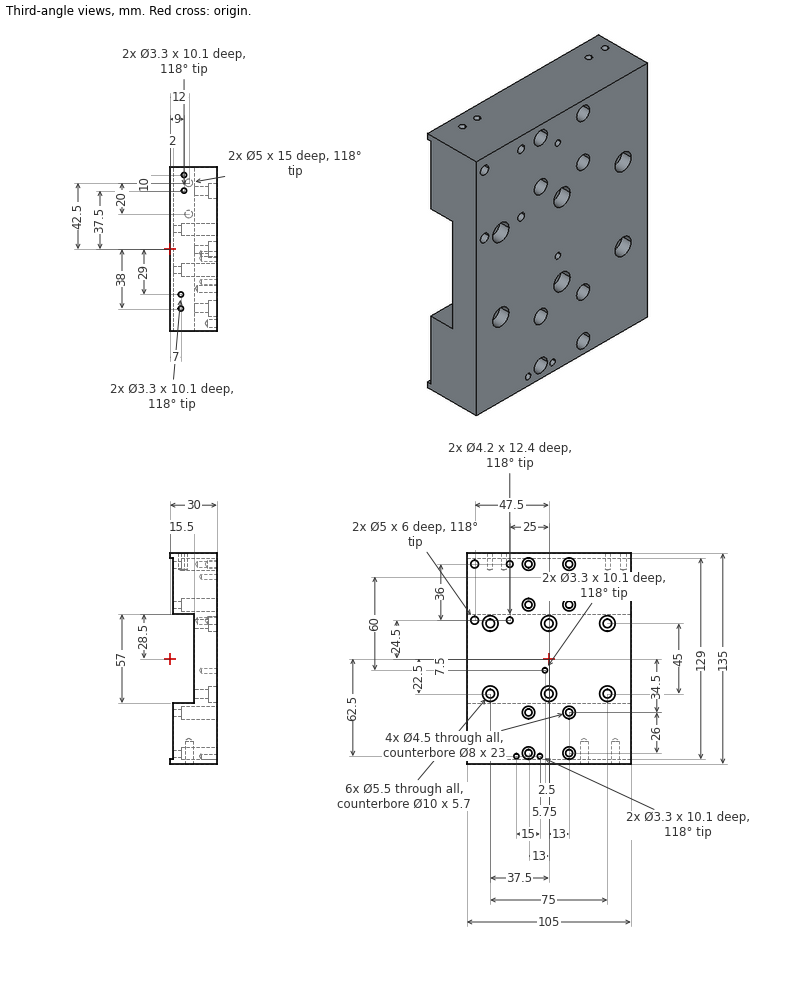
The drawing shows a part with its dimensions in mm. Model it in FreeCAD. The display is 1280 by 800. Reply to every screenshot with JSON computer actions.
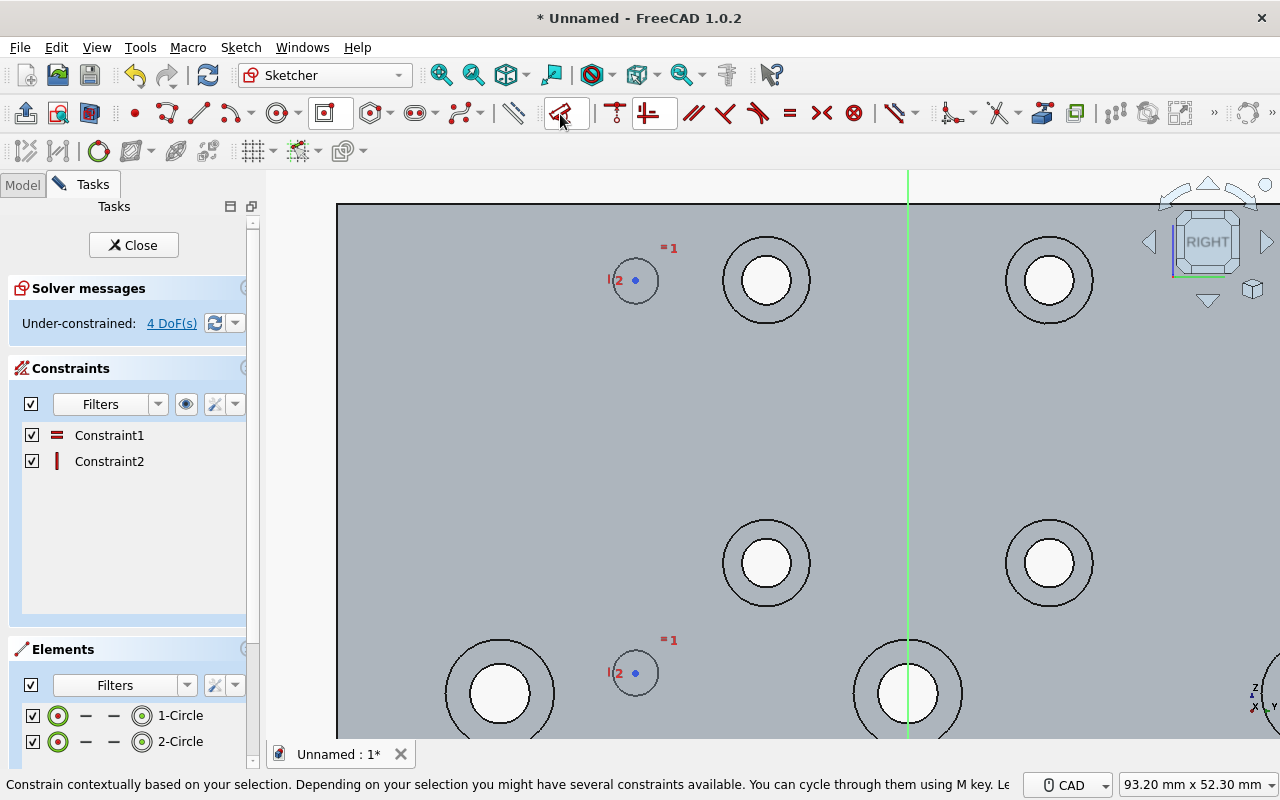
{"action": "left_click", "coordinate": [652, 657]}
{"action": "left_click", "coordinate": [675, 634]}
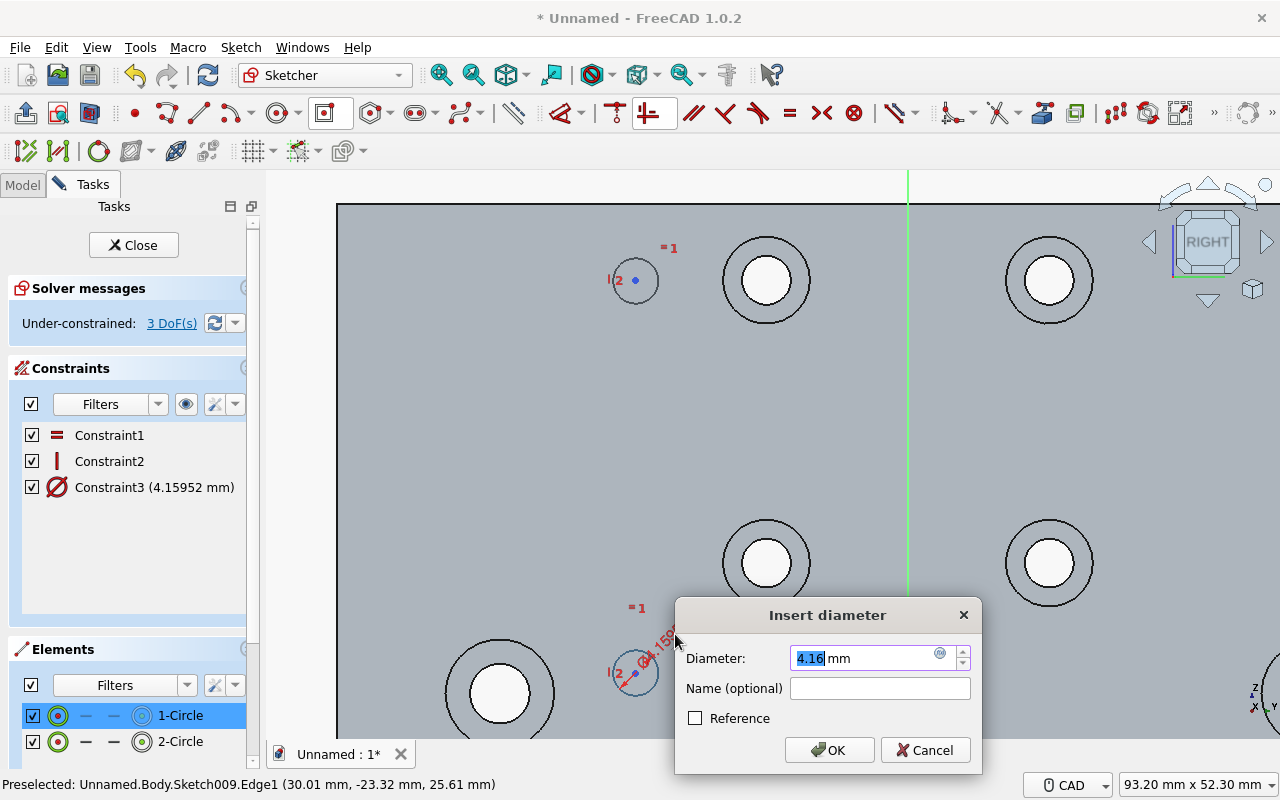
{"action": "type", "text": "4.2"}
{"action": "key", "text": "Return"}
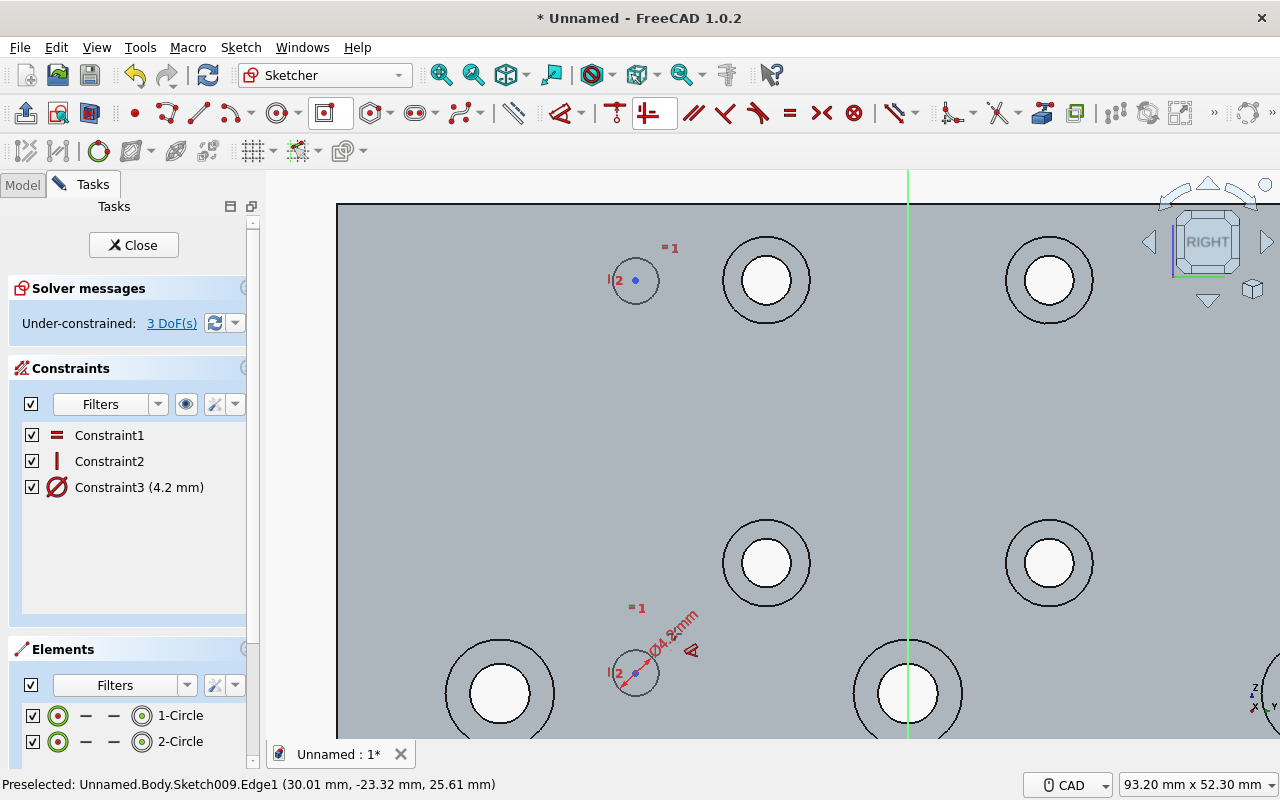
{"action": "left_click", "coordinate": [636, 673]}
{"action": "left_click", "coordinate": [772, 639]}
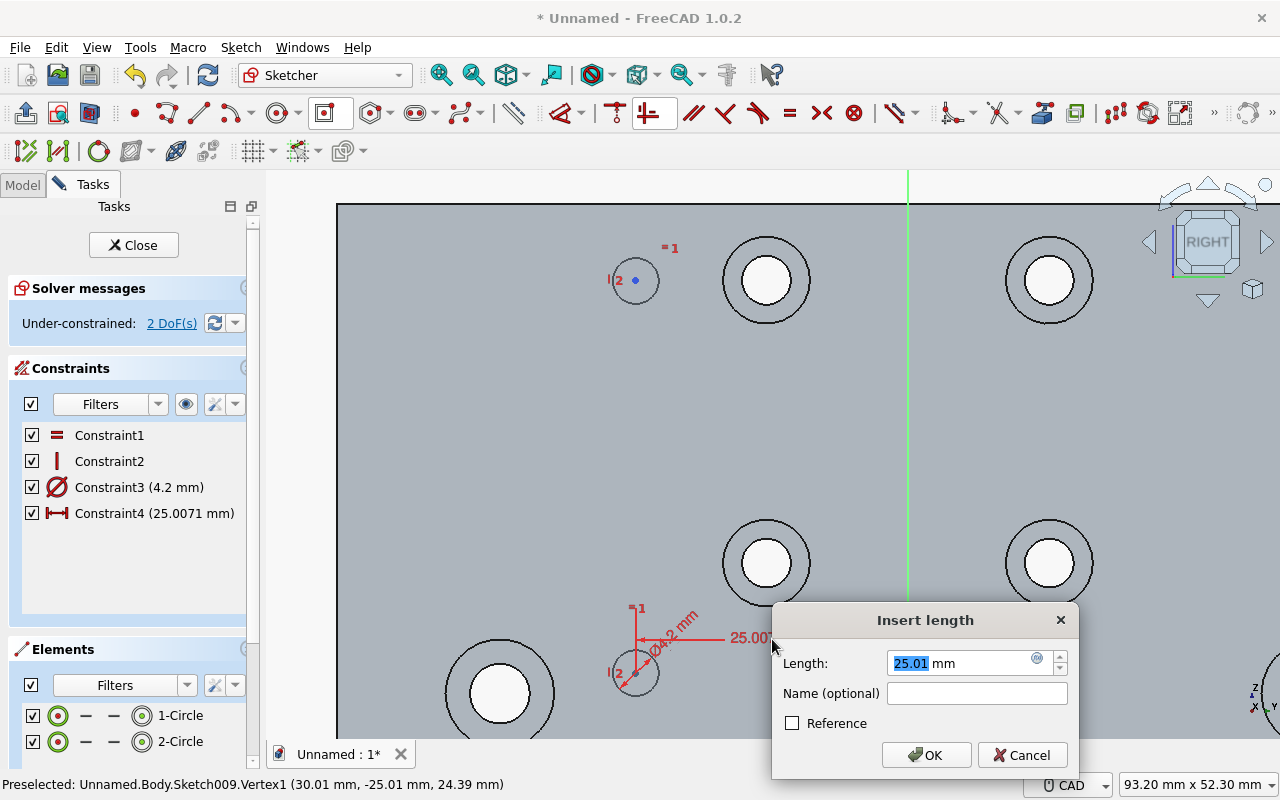
{"action": "type", "text": "25"}
{"action": "key", "text": "Return"}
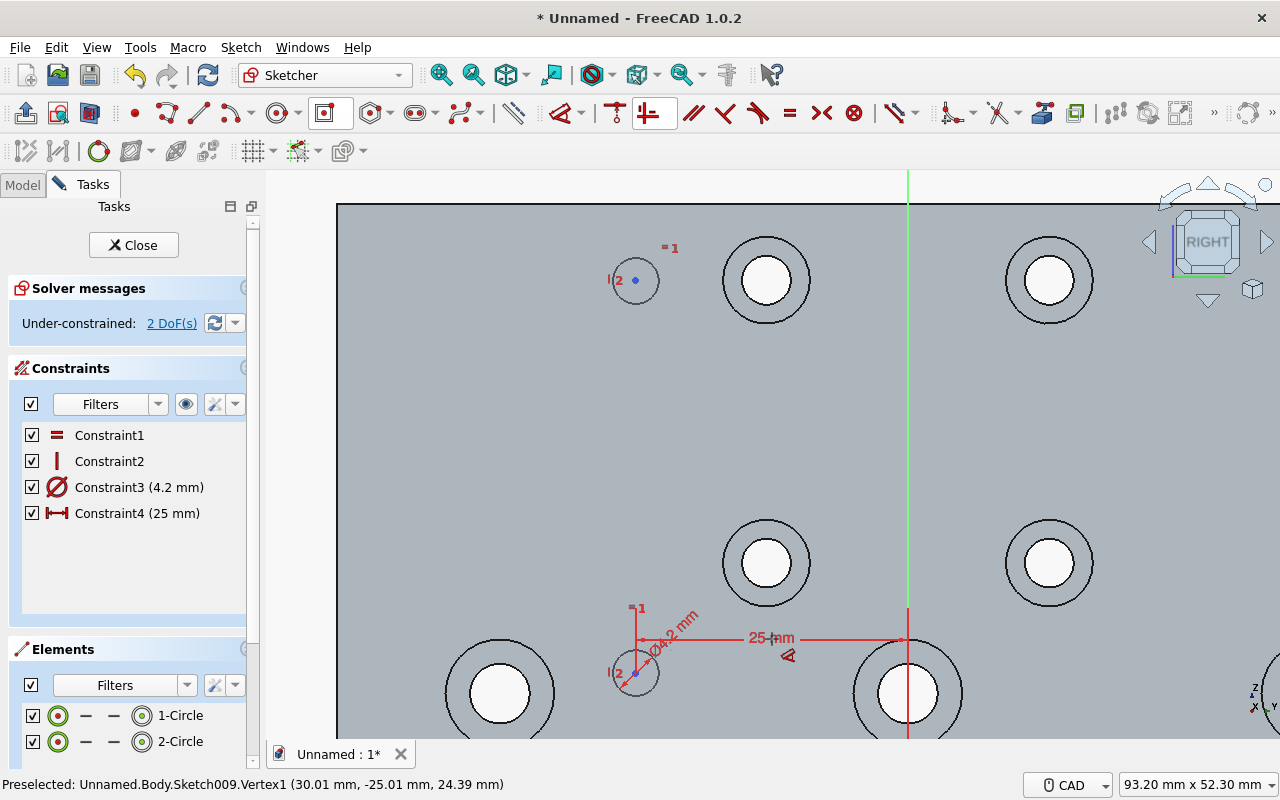
{"action": "left_click", "coordinate": [636, 673]}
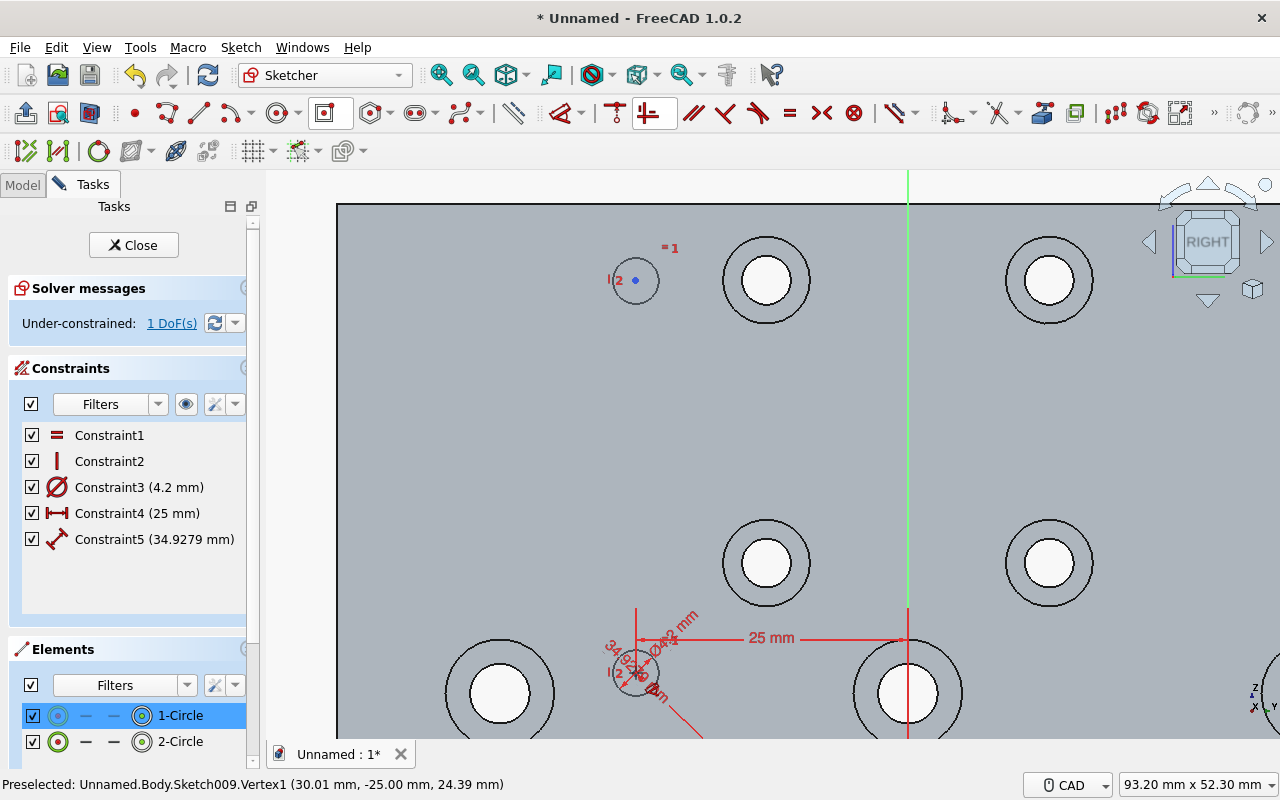
{"action": "left_click", "coordinate": [636, 281]}
{"action": "left_click", "coordinate": [602, 477]}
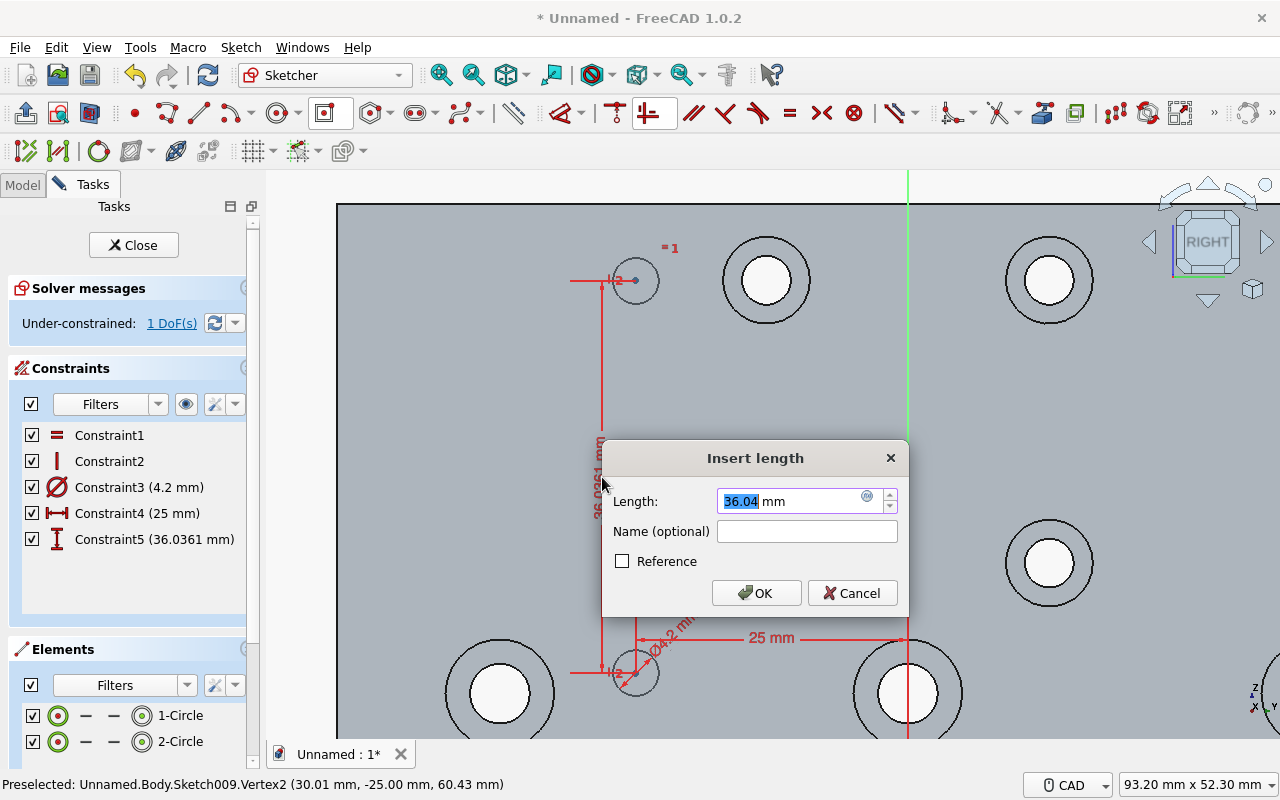
{"action": "type", "text": "36"}
{"action": "key", "text": "Return"}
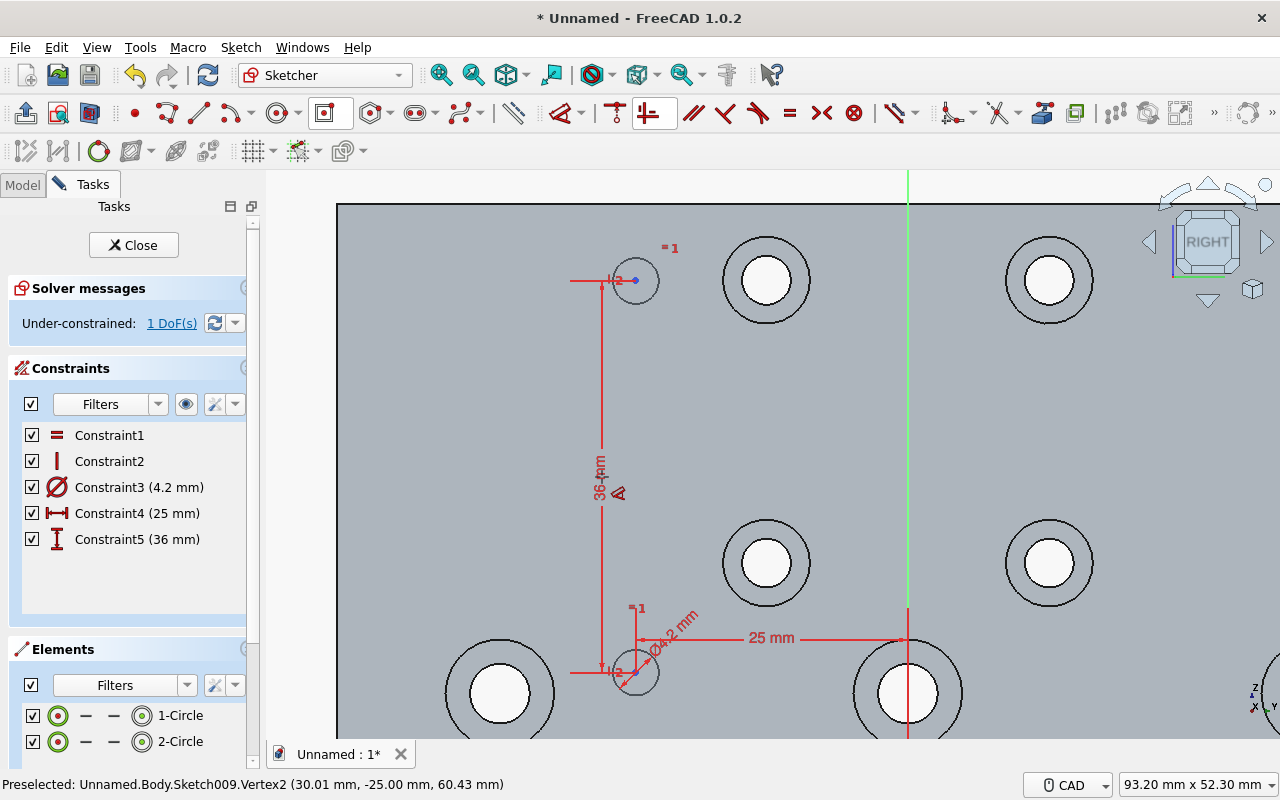
{"action": "left_click", "coordinate": [636, 673]}
{"action": "left_click", "coordinate": [942, 692]}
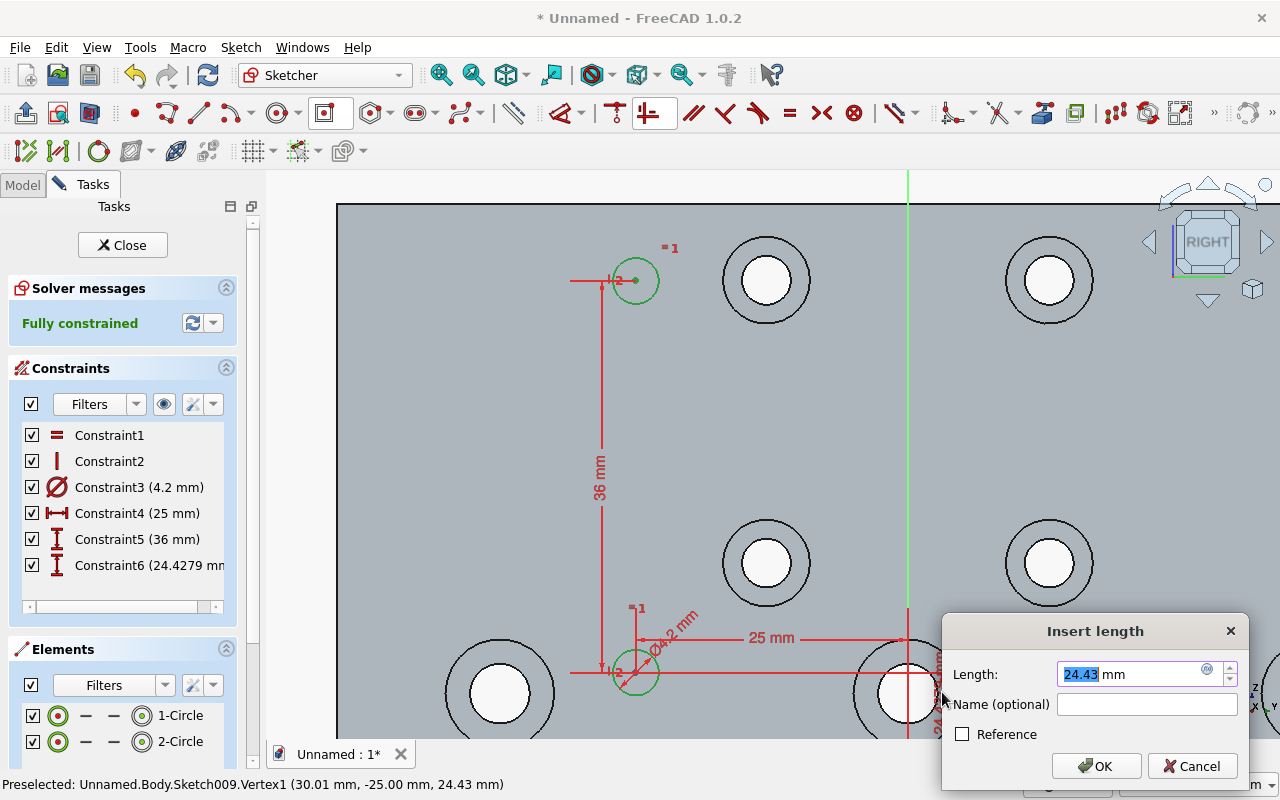
{"action": "type", "text": "24.5"}
{"action": "key", "text": "Return"}
{"action": "key", "text": "Escape"}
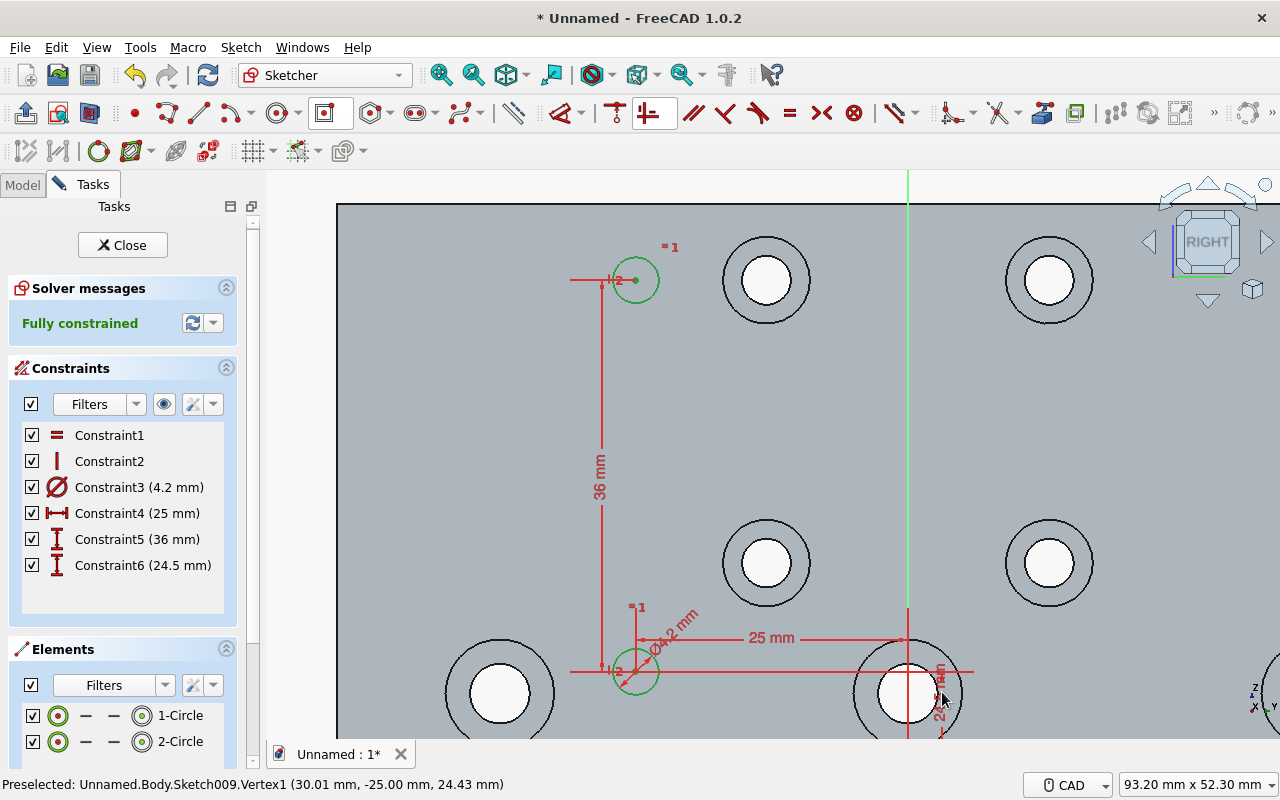
{"action": "left_click", "coordinate": [123, 245]}